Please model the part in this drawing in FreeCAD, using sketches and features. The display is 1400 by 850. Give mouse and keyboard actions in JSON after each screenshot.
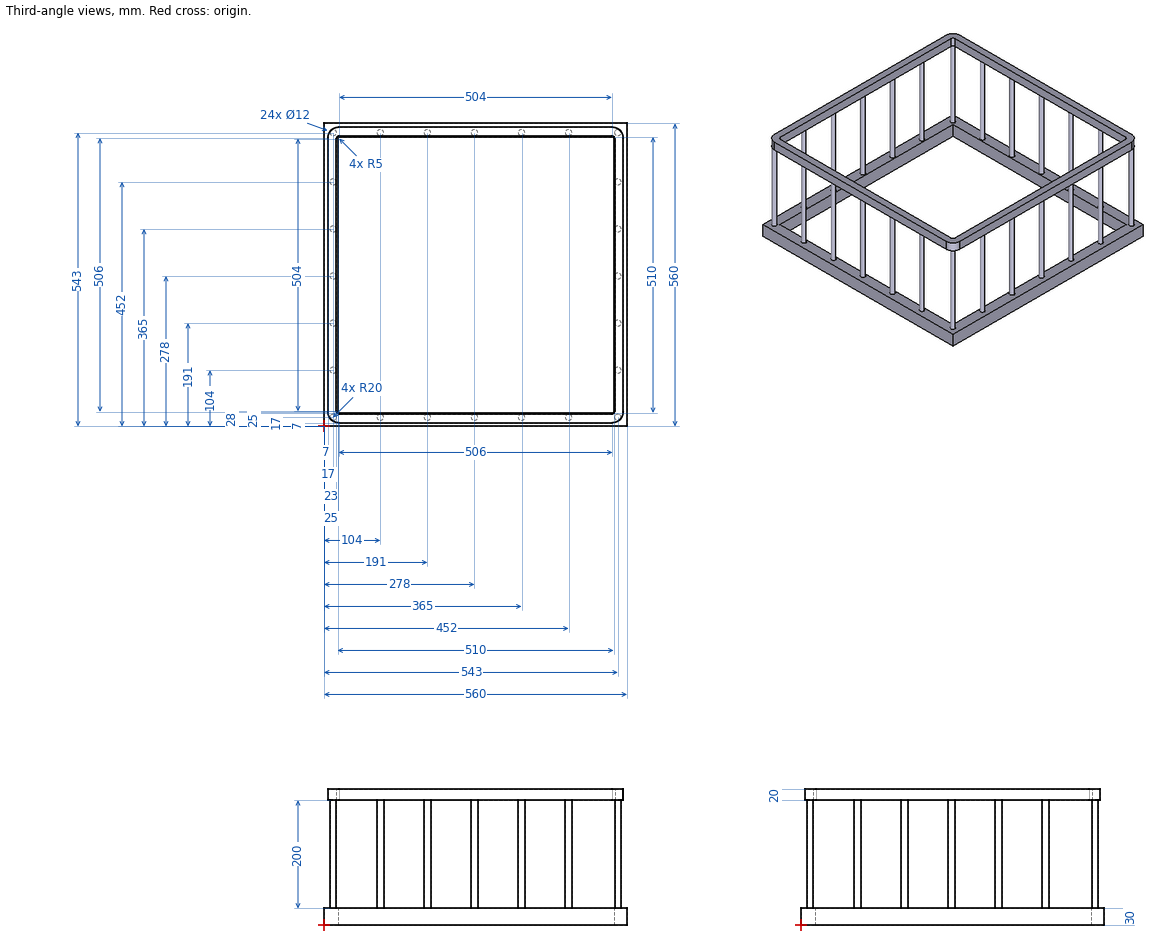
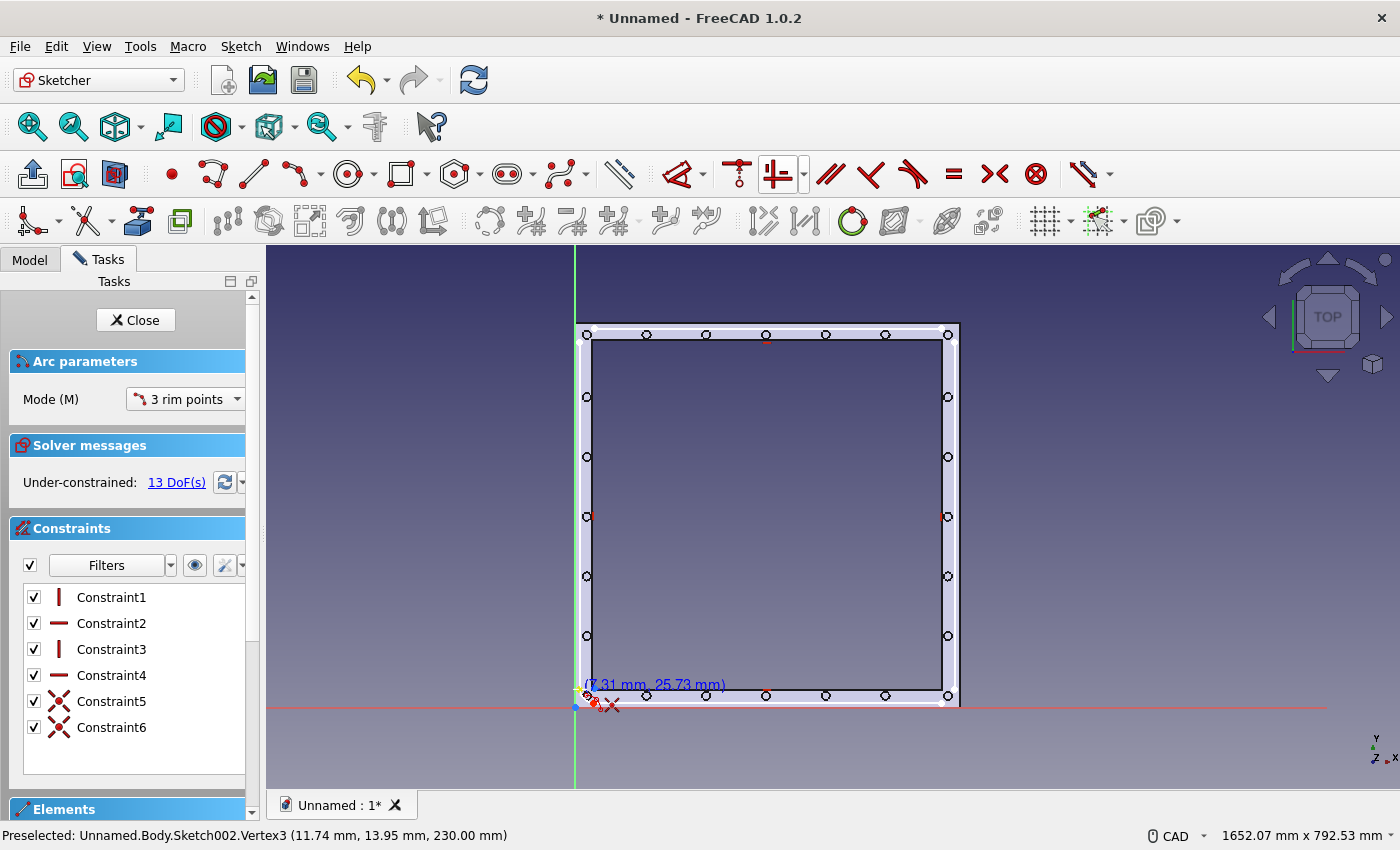
{"action": "scroll", "coordinate": [941, 703], "scroll_direction": "up", "scroll_amount": 6}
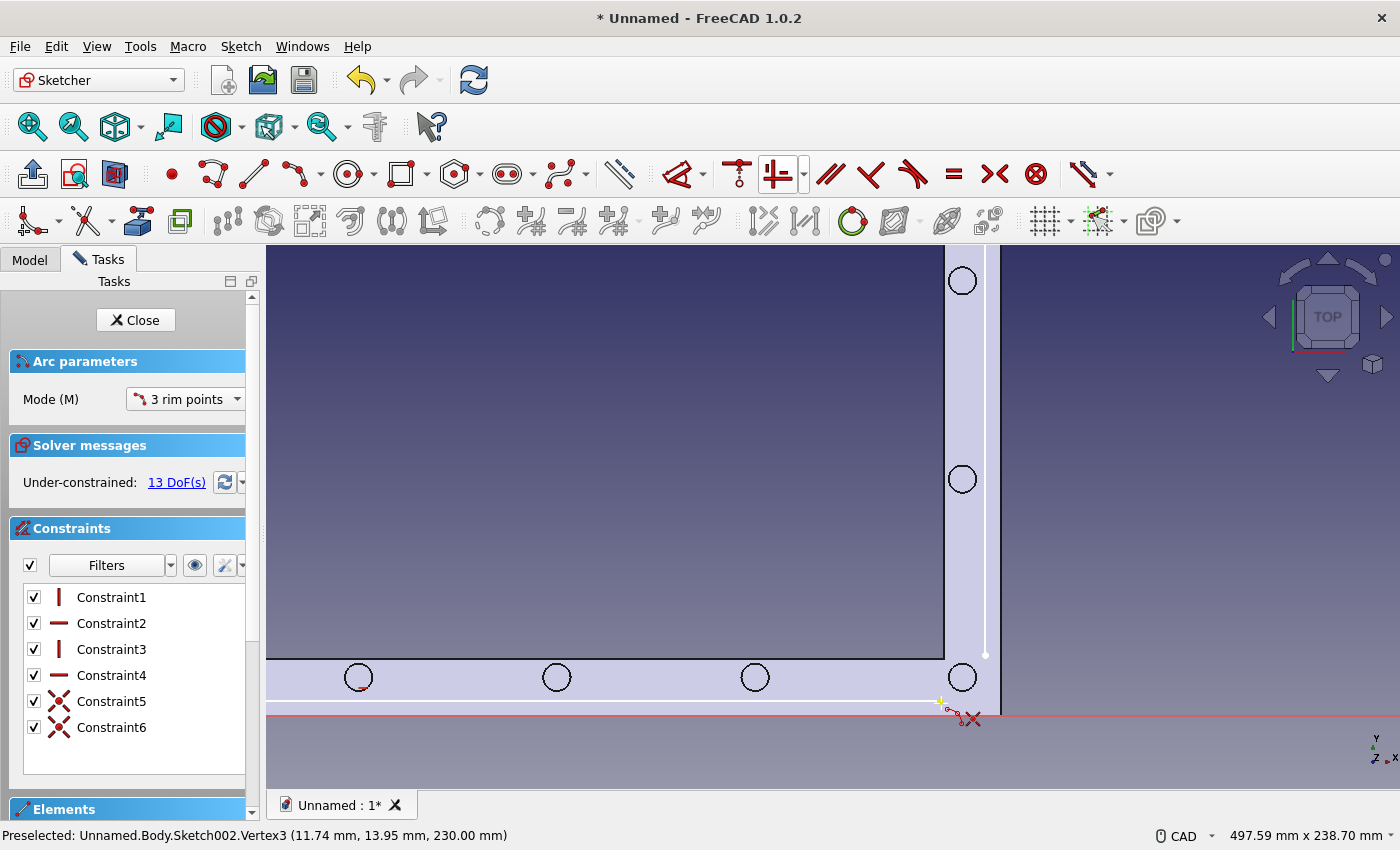
{"action": "left_click", "coordinate": [940, 701]}
{"action": "left_click", "coordinate": [985, 656]}
{"action": "left_click", "coordinate": [972, 687]}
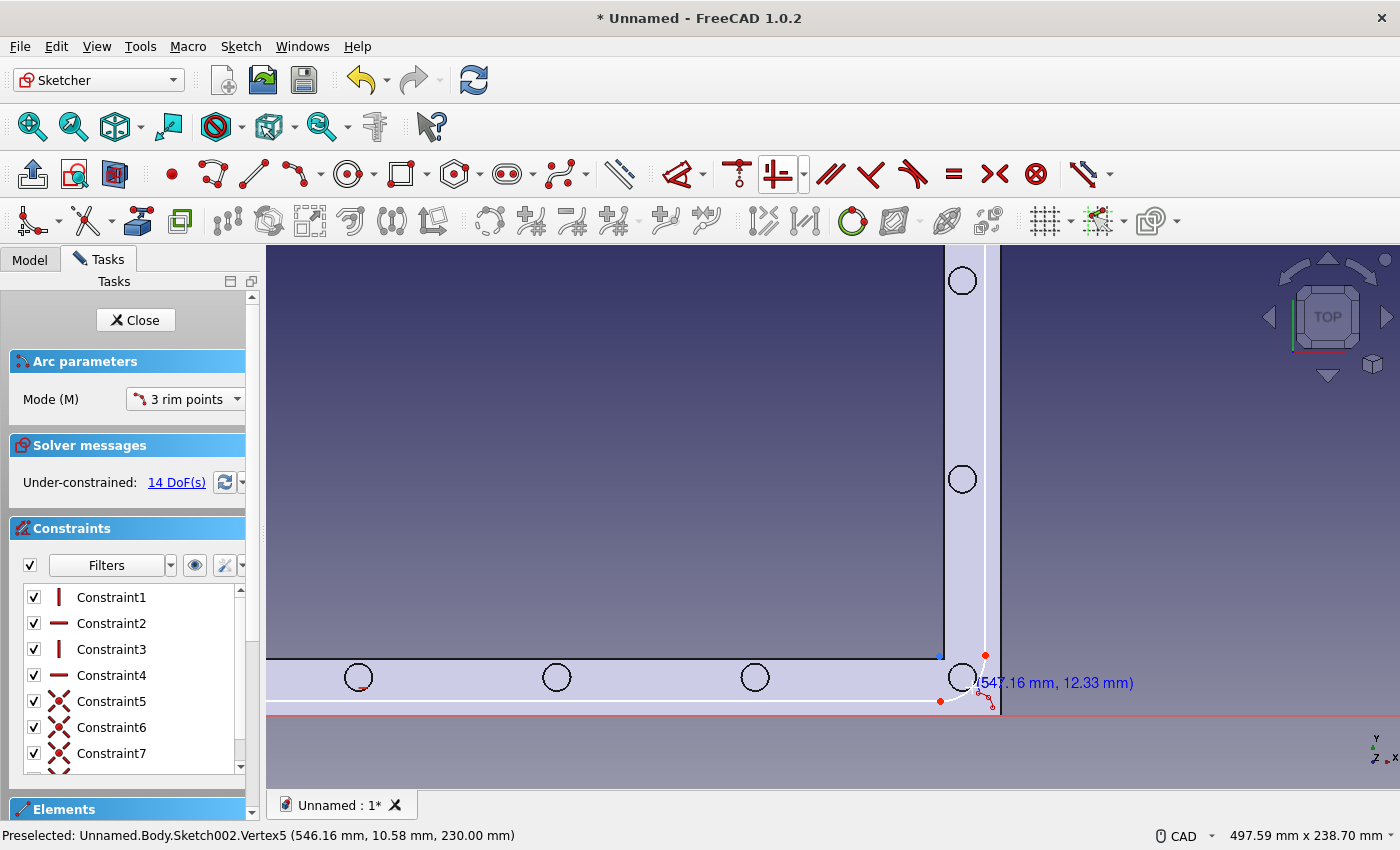
{"action": "scroll", "coordinate": [941, 703], "scroll_direction": "down", "scroll_amount": 6}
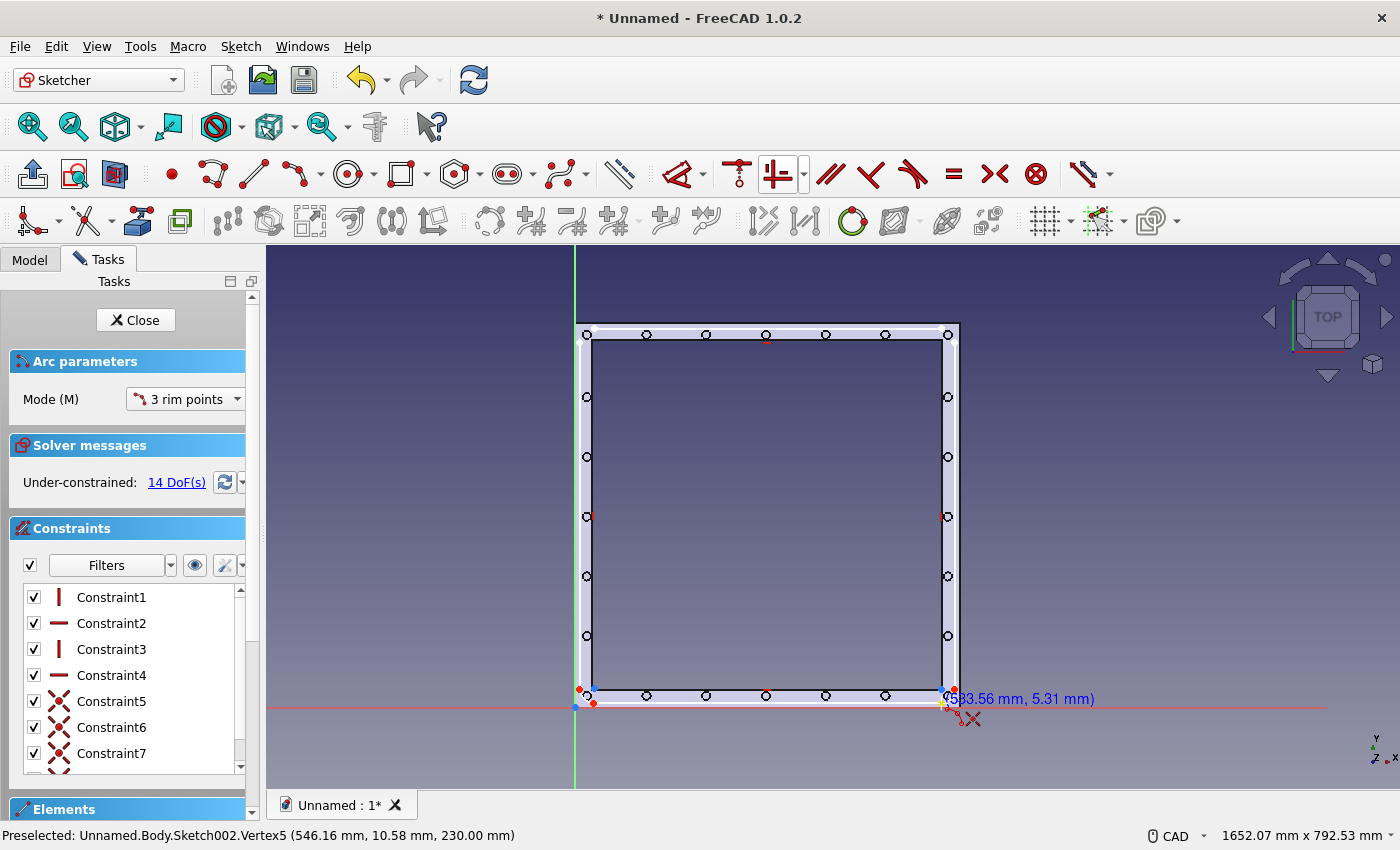
{"action": "left_click", "coordinate": [955, 343]}
{"action": "left_click", "coordinate": [941, 329]}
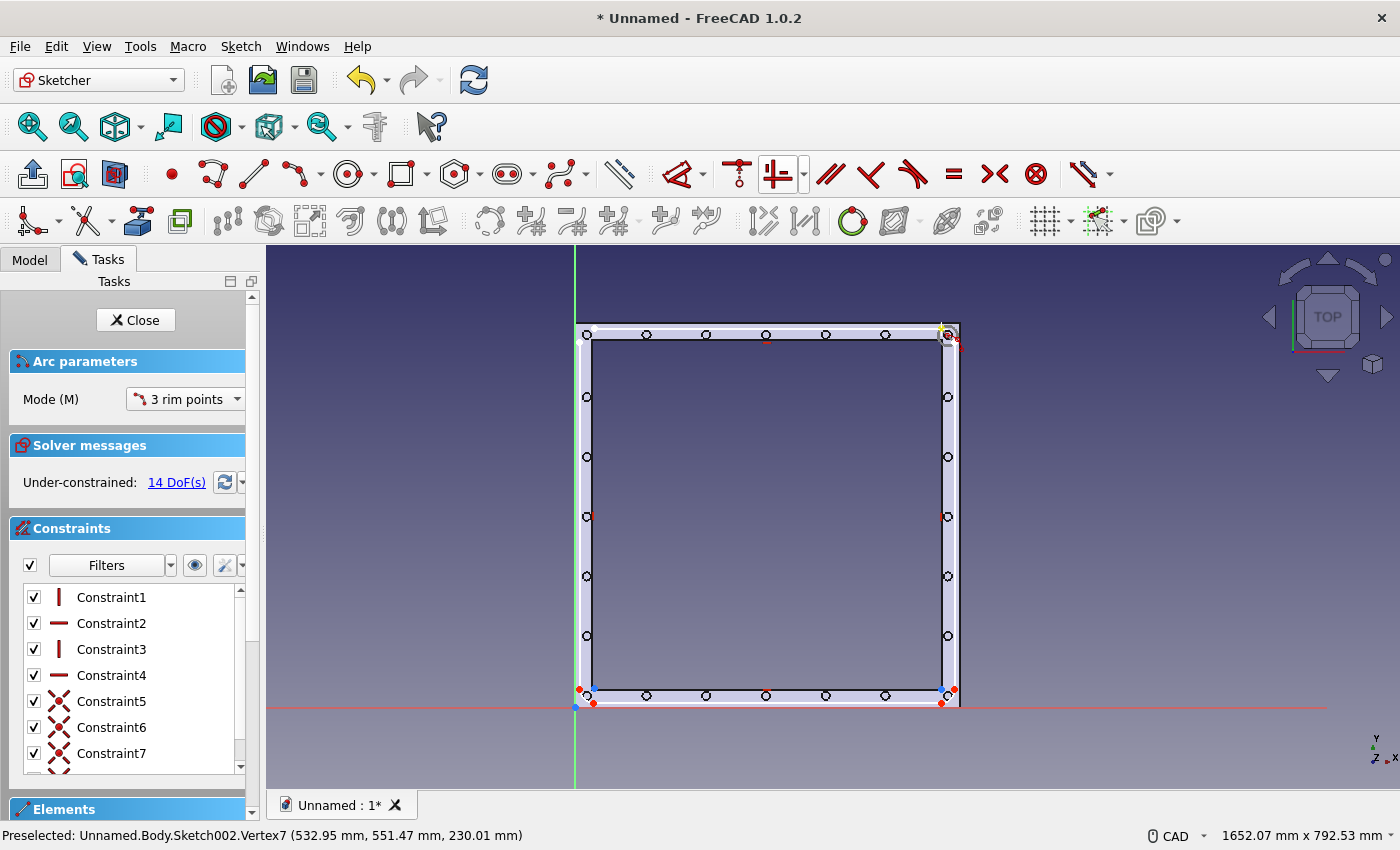
{"action": "scroll", "coordinate": [951, 332], "scroll_direction": "up", "scroll_amount": 7}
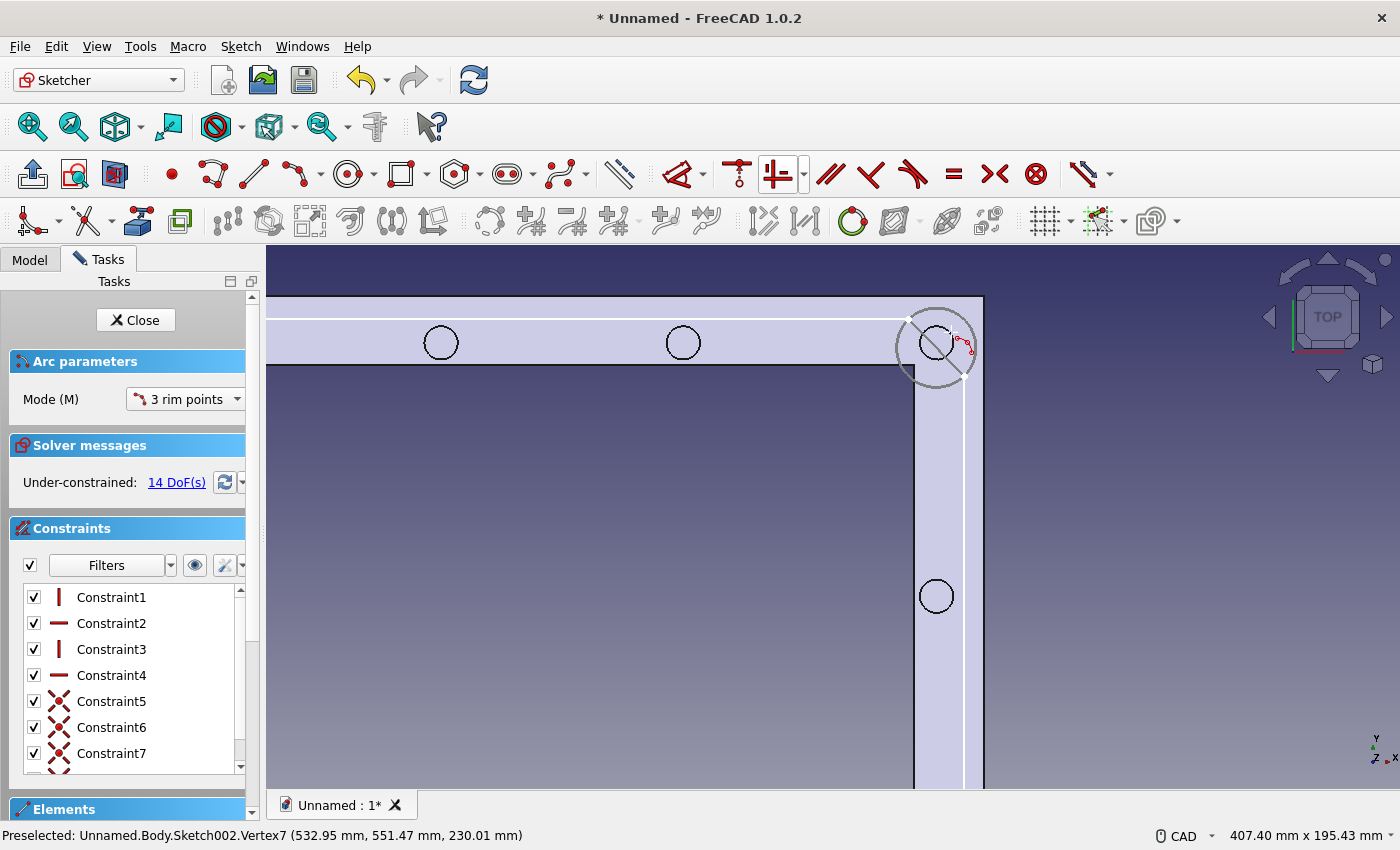
{"action": "left_click", "coordinate": [948, 331]}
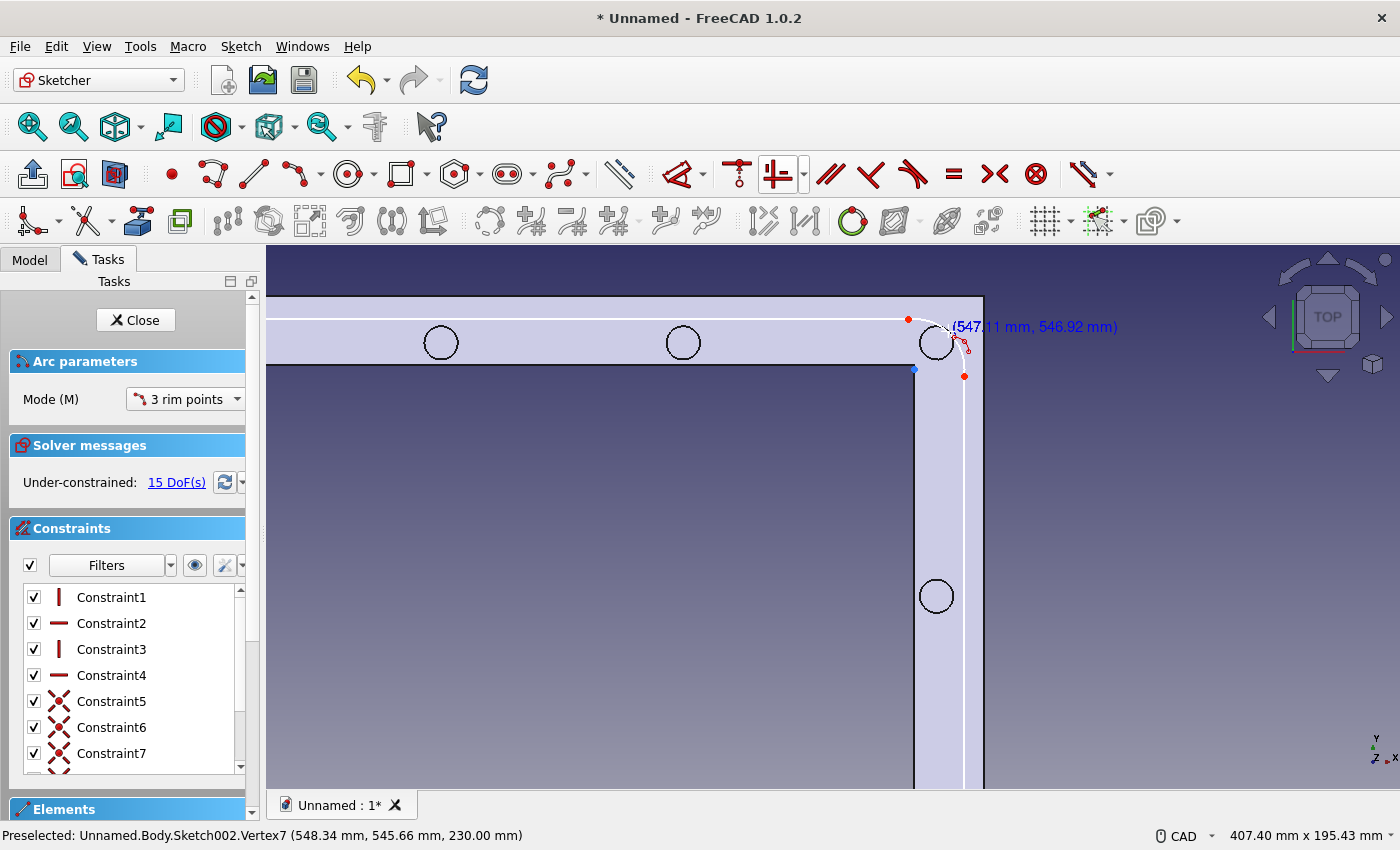
{"action": "scroll", "coordinate": [951, 331], "scroll_direction": "down", "scroll_amount": 7}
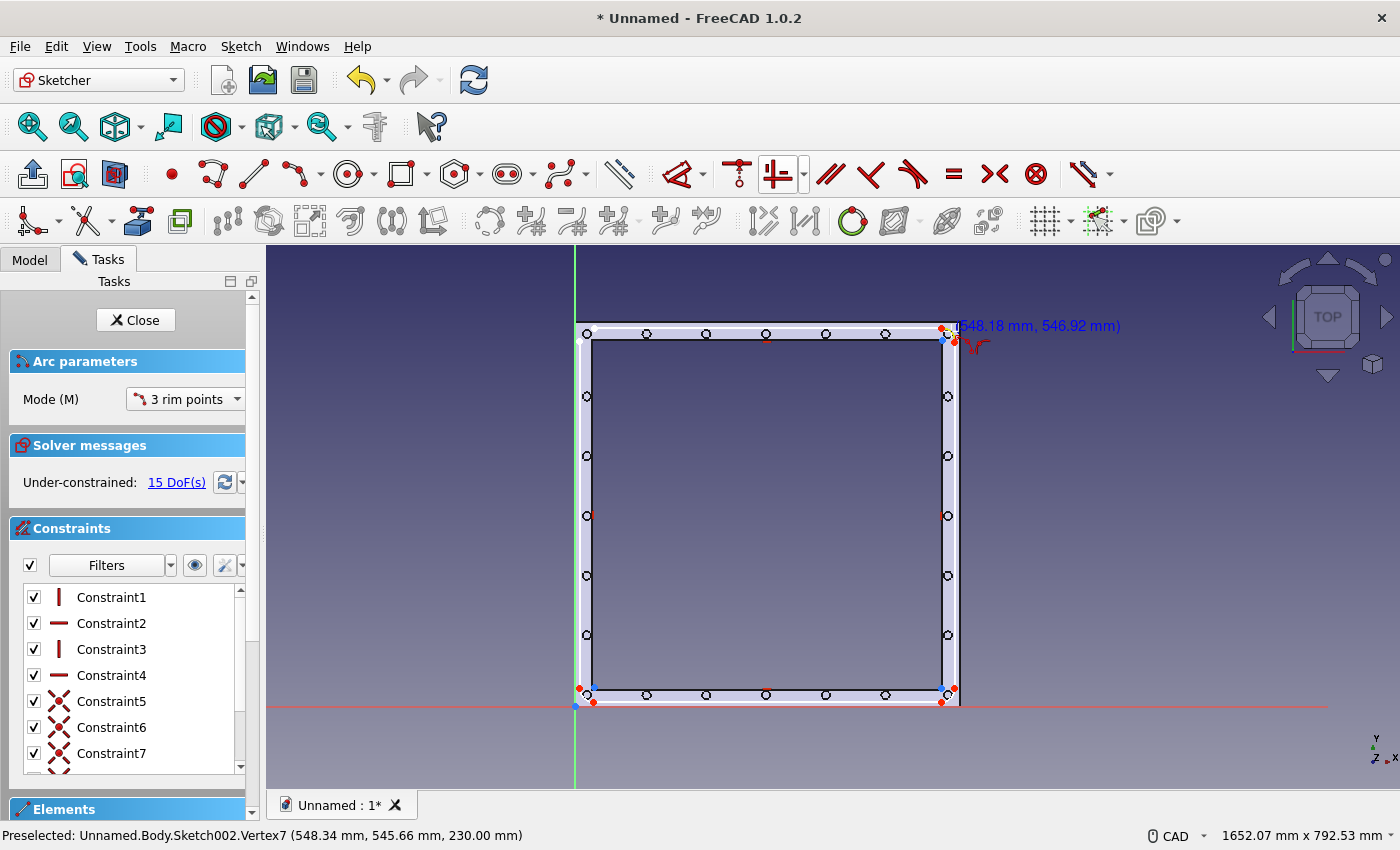
{"action": "left_click", "coordinate": [594, 328]}